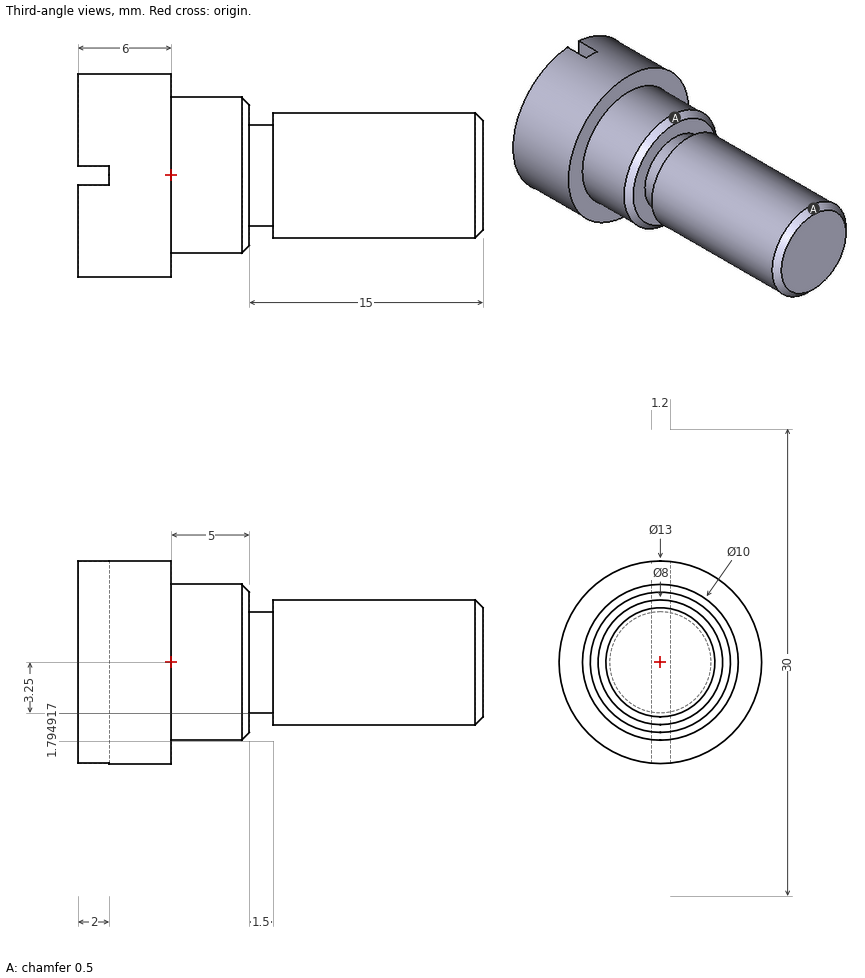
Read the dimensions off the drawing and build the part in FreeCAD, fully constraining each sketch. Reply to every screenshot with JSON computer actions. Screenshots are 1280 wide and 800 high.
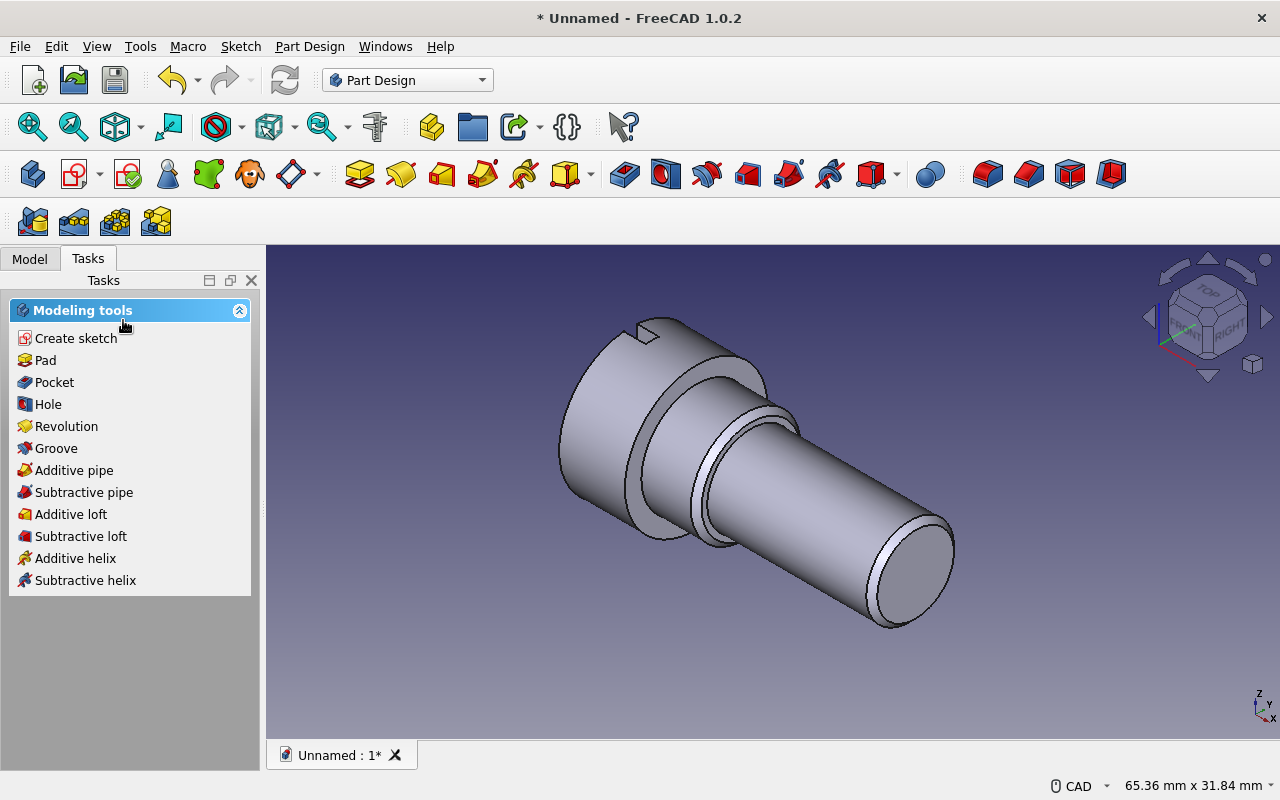
{"action": "left_click", "coordinate": [707, 174]}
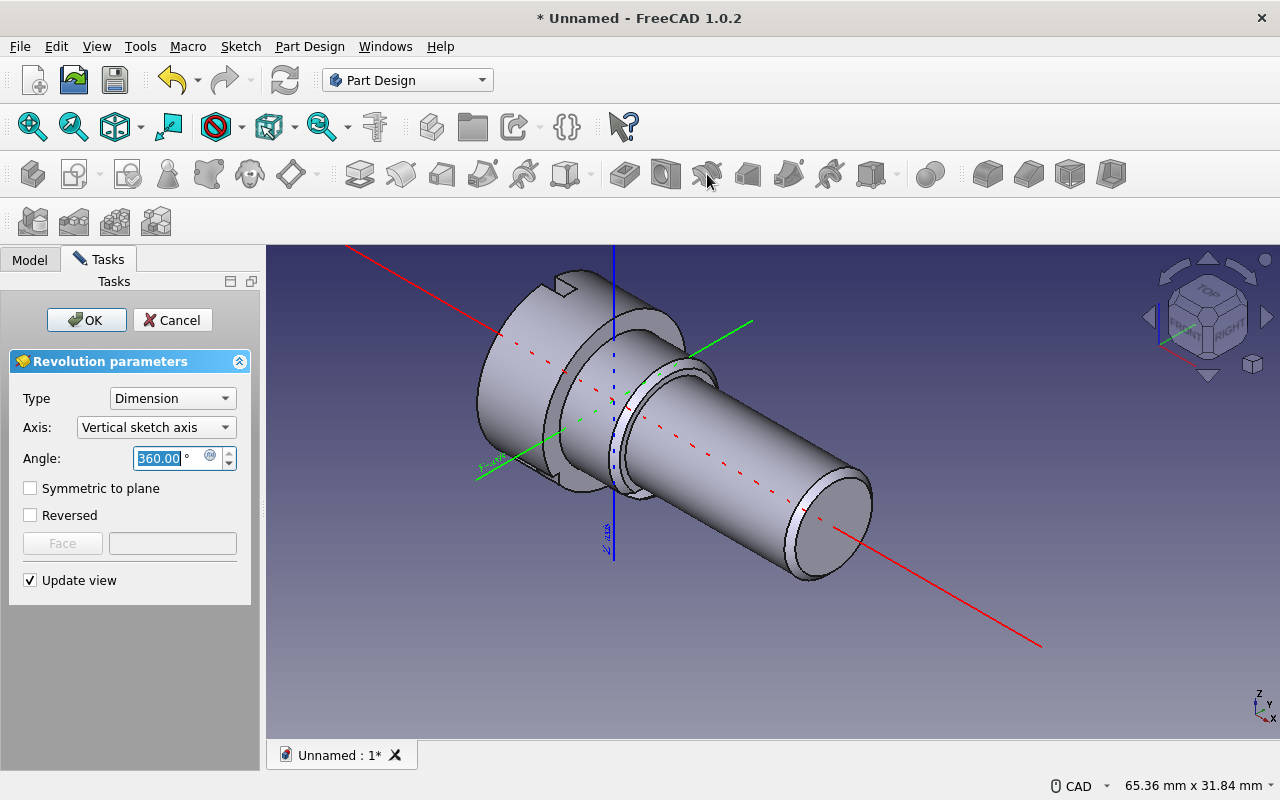
{"action": "left_click", "coordinate": [157, 428]}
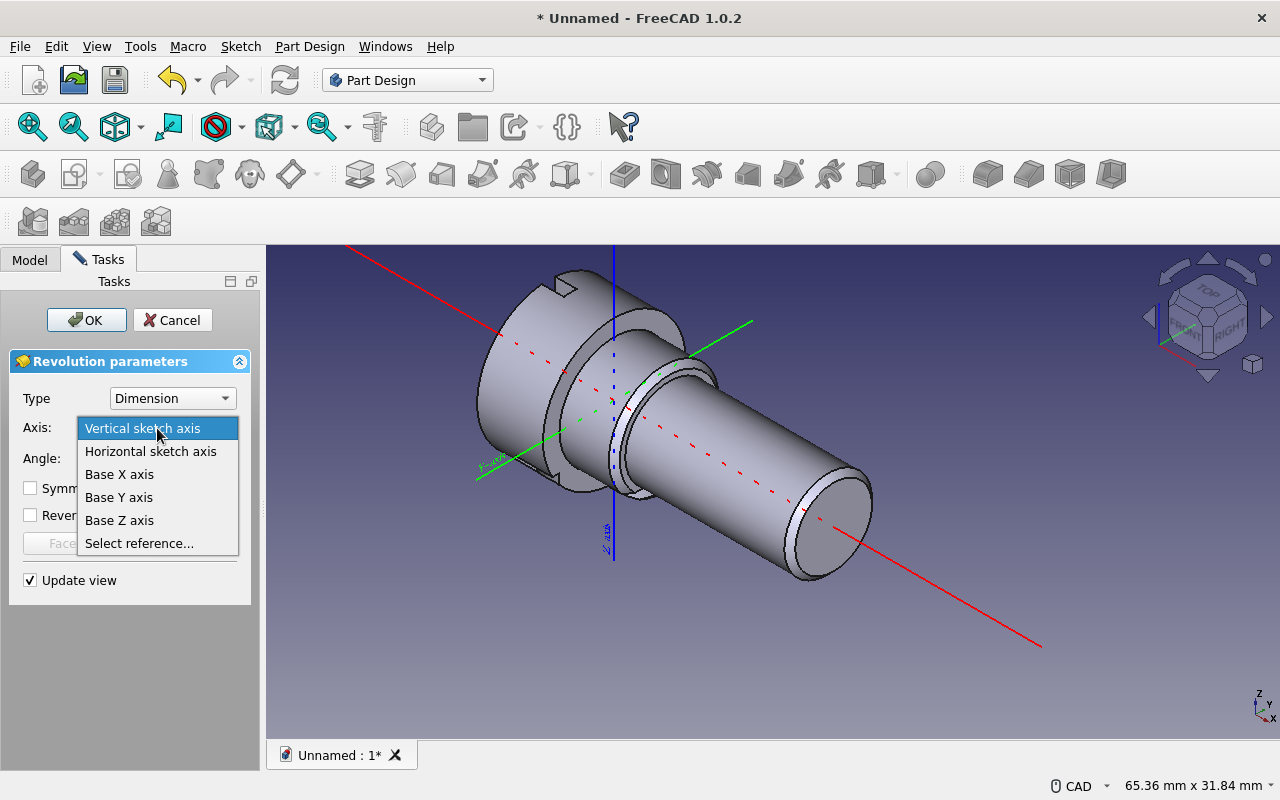
{"action": "left_click", "coordinate": [156, 452]}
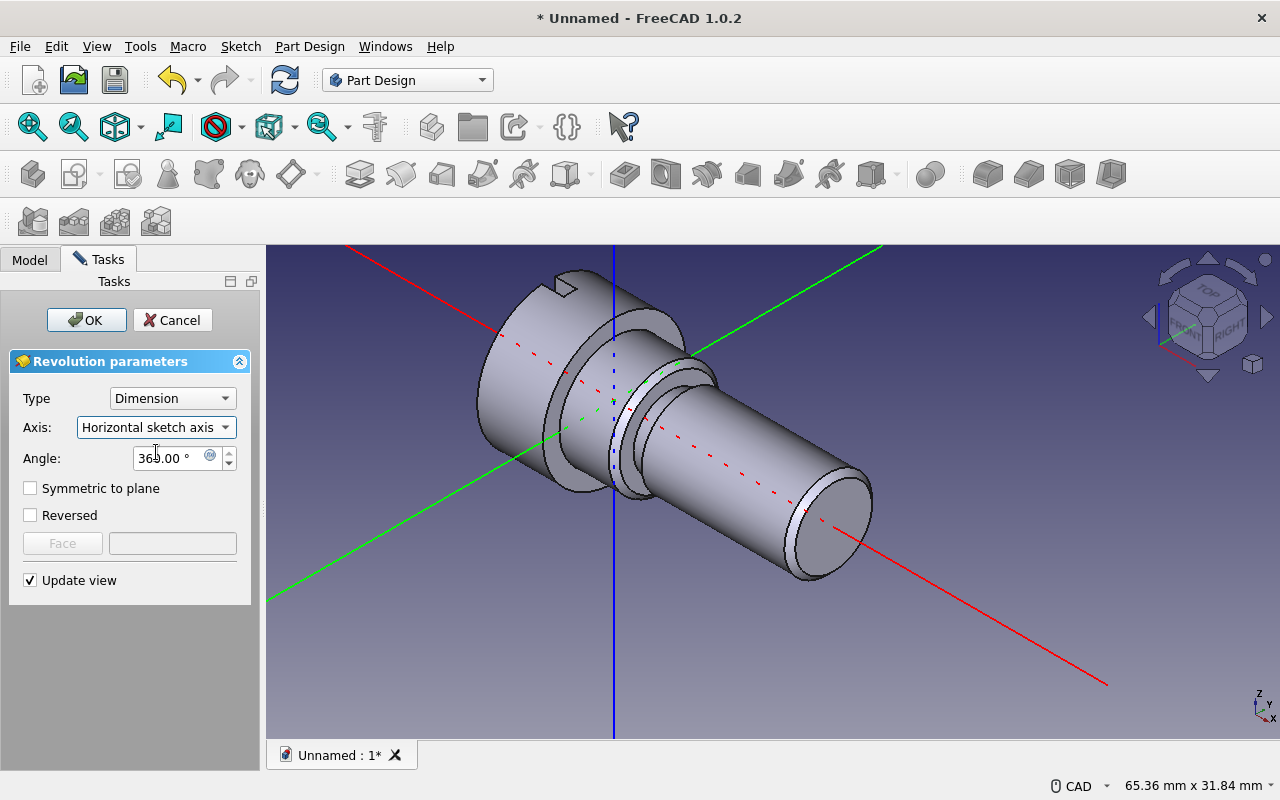
{"action": "left_click", "coordinate": [87, 320]}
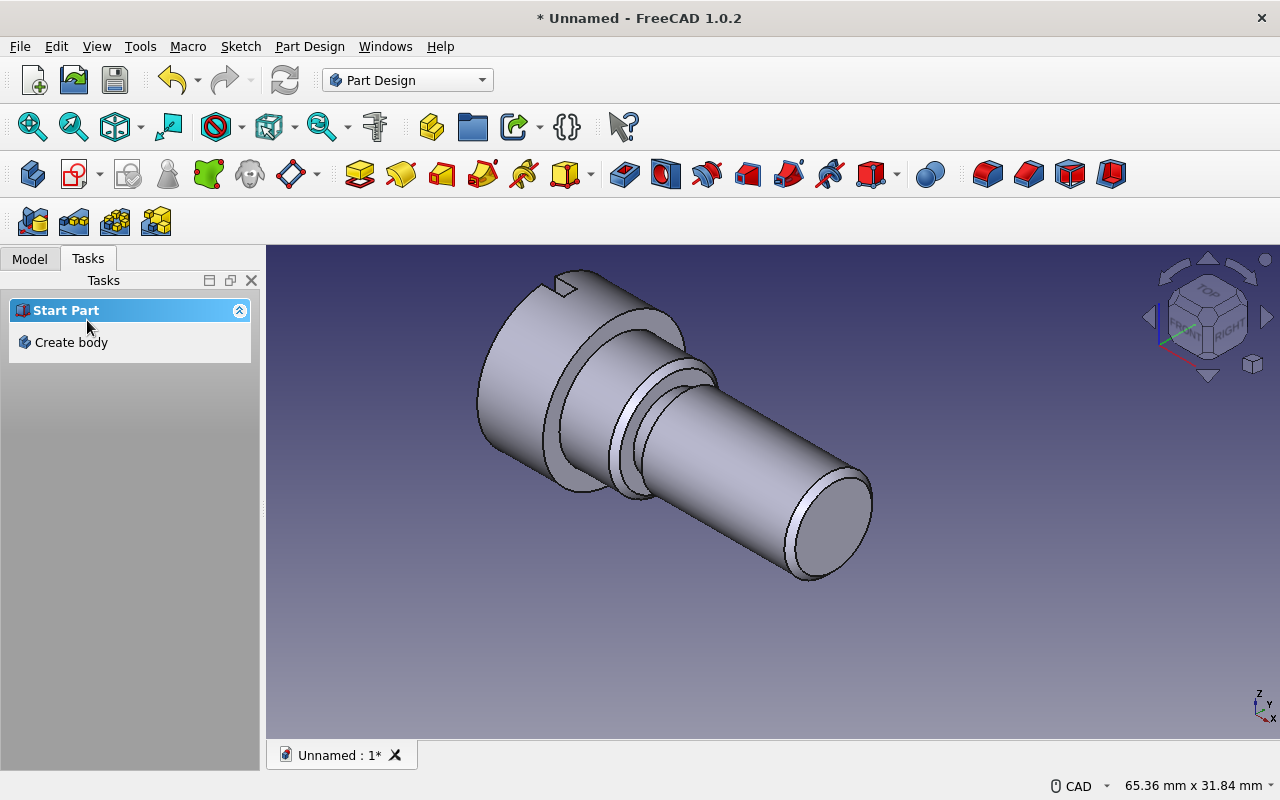
{"action": "left_click", "coordinate": [33, 128]}